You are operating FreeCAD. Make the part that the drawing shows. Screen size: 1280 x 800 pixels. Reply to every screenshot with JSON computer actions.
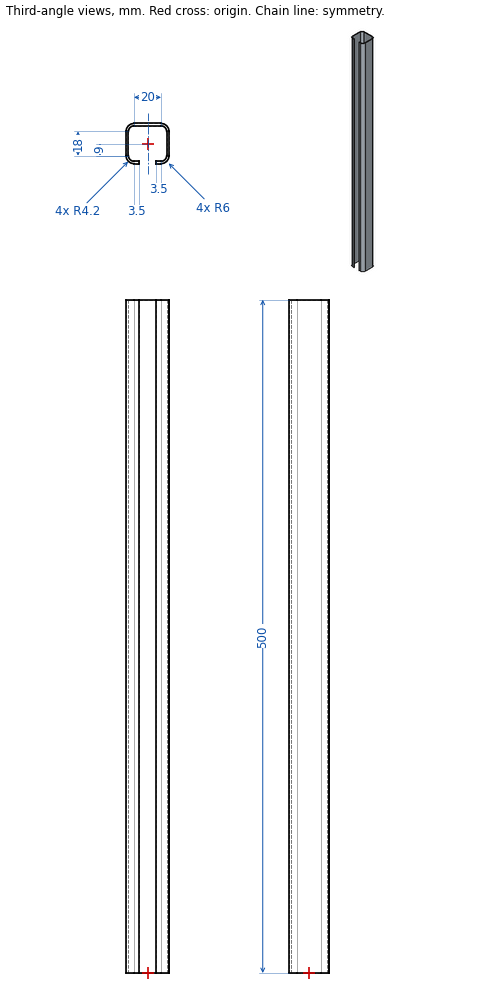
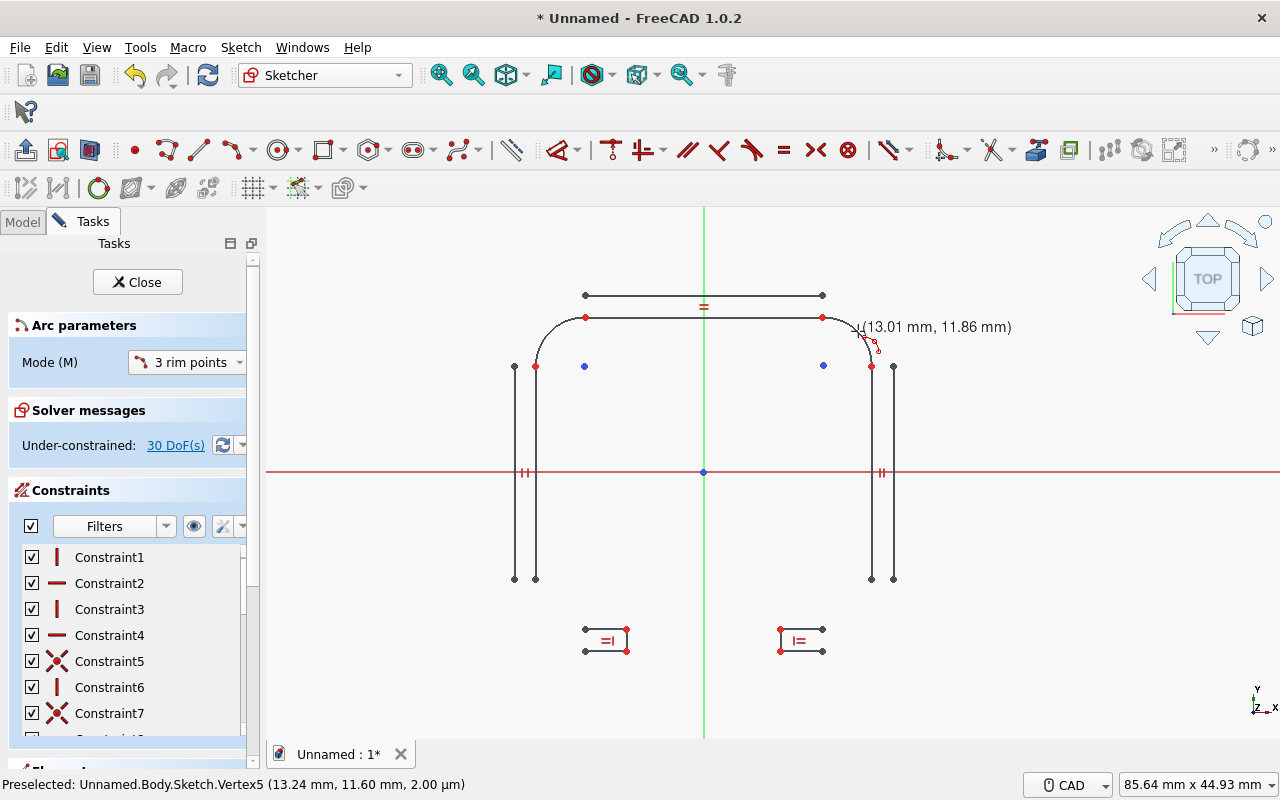
{"action": "left_click", "coordinate": [872, 580]}
{"action": "left_click", "coordinate": [823, 629]}
{"action": "left_click", "coordinate": [858, 614]}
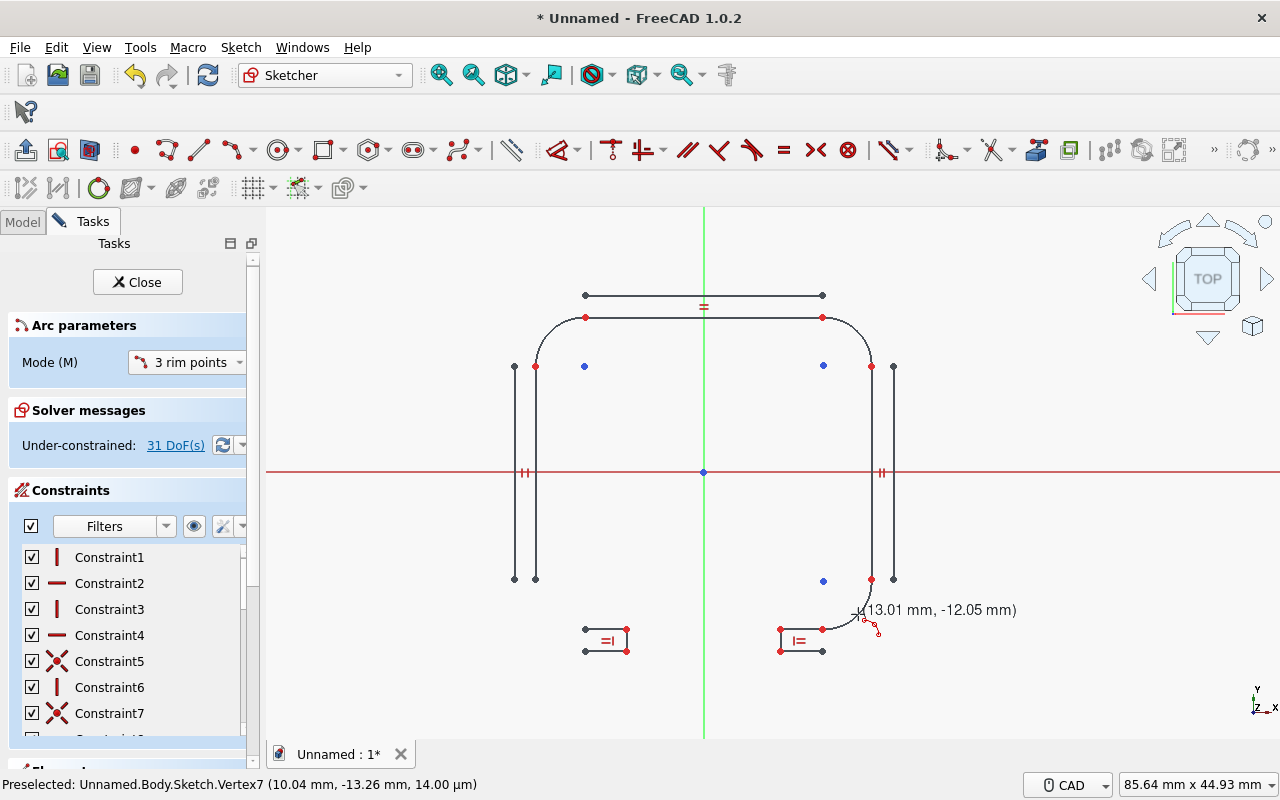
{"action": "left_click", "coordinate": [823, 651]}
{"action": "left_click", "coordinate": [894, 580]}
{"action": "left_click", "coordinate": [873, 629]}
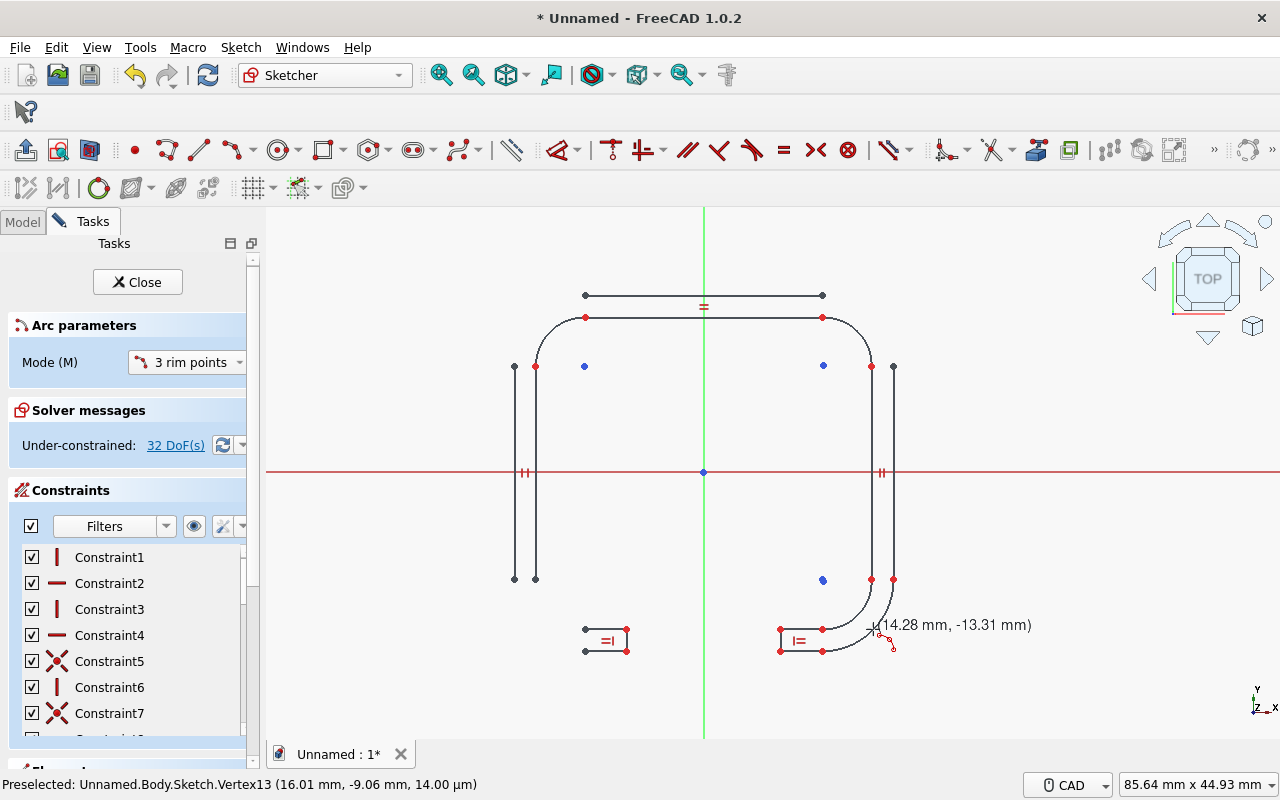
{"action": "left_click", "coordinate": [894, 366]}
{"action": "left_click", "coordinate": [823, 296]}
{"action": "left_click", "coordinate": [873, 316]}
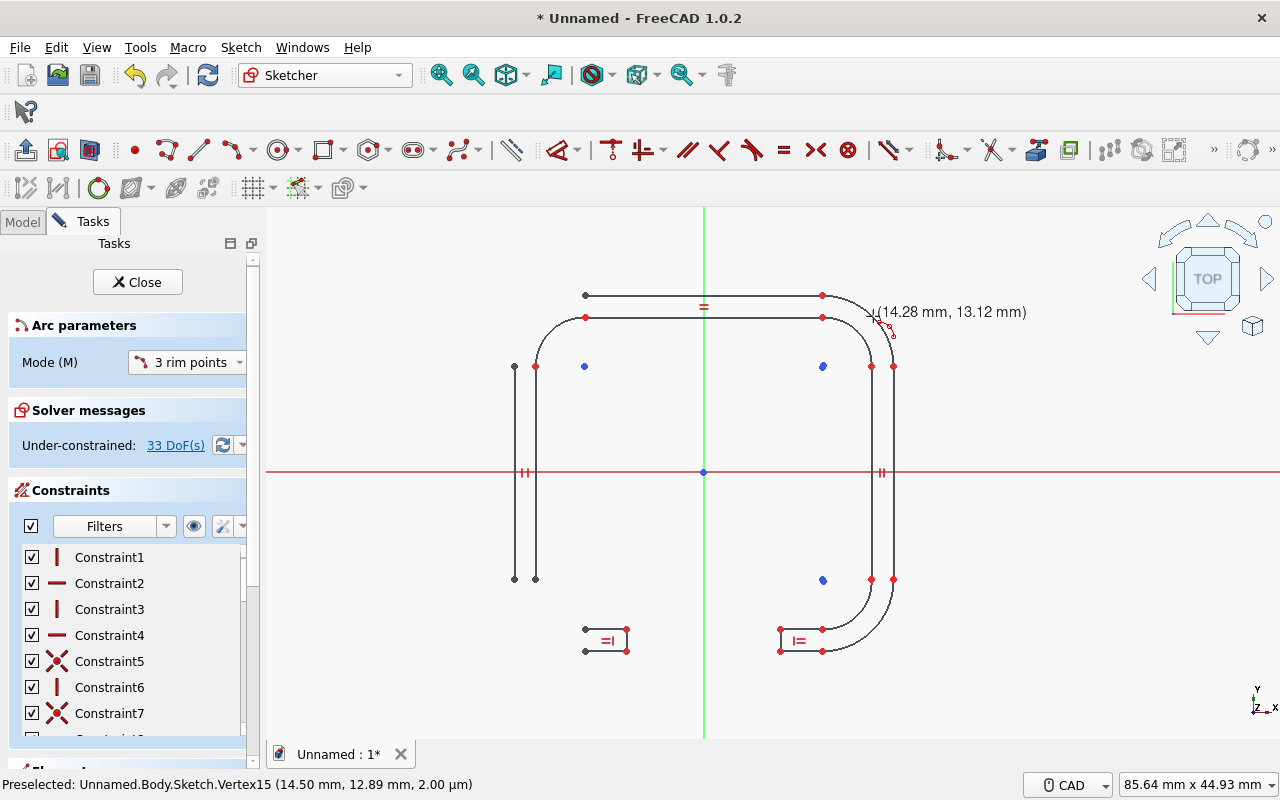
{"action": "left_click", "coordinate": [586, 296]}
{"action": "left_click", "coordinate": [515, 366]}
{"action": "left_click", "coordinate": [535, 316]}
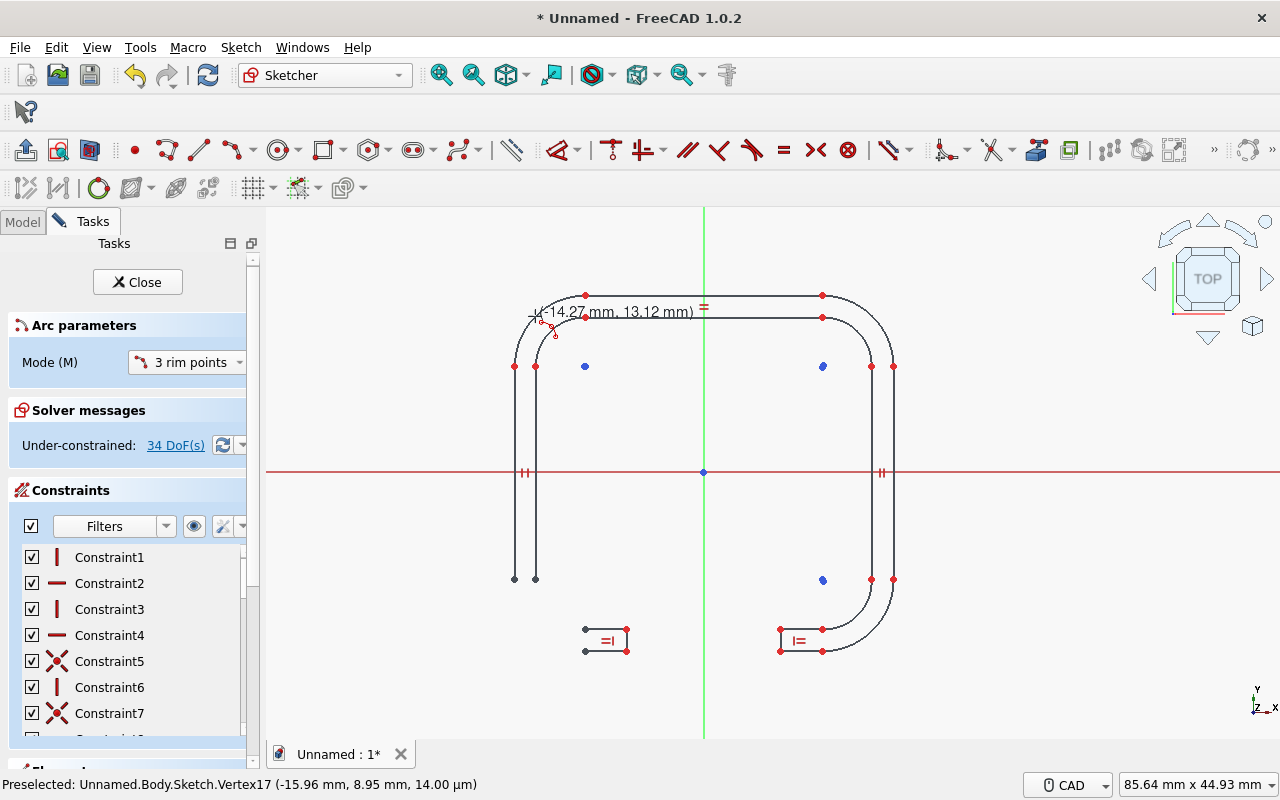
{"action": "left_click", "coordinate": [515, 580]}
{"action": "left_click", "coordinate": [586, 651]}
{"action": "left_click", "coordinate": [535, 629]}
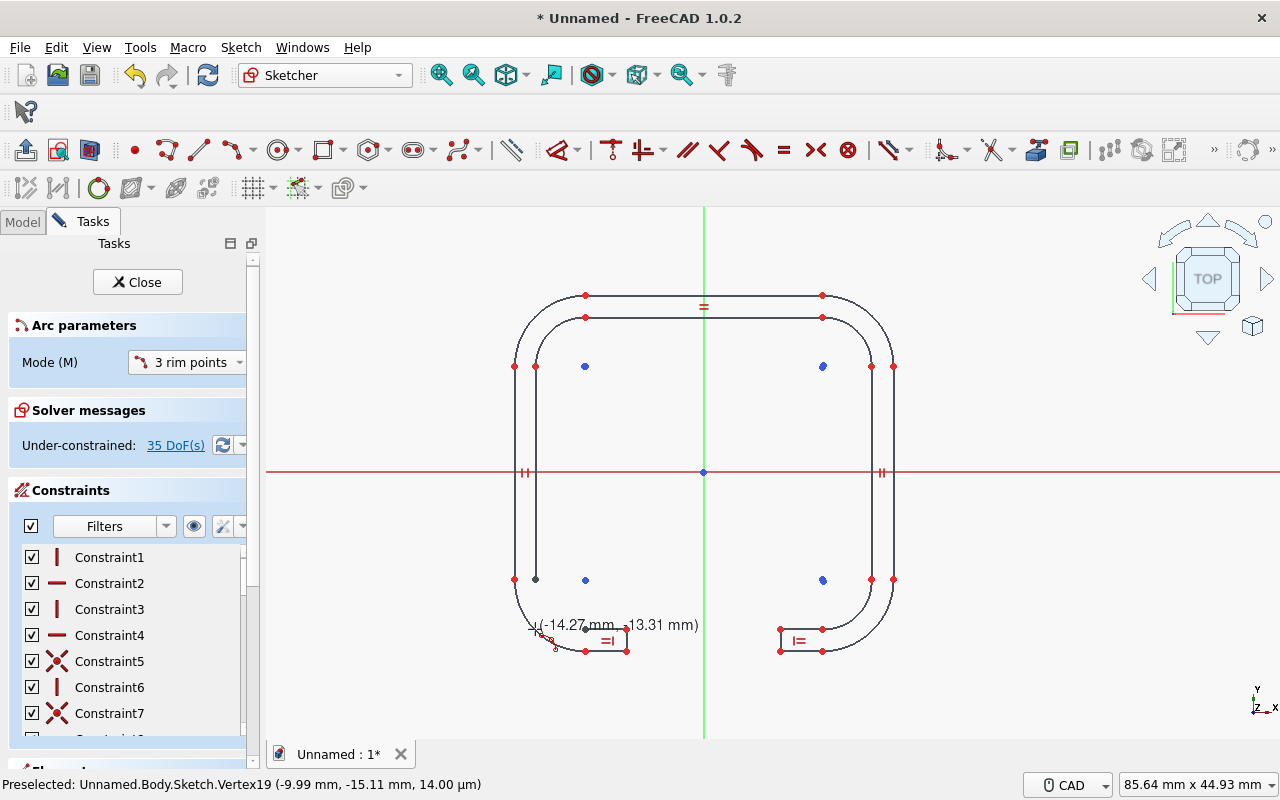
{"action": "left_click", "coordinate": [586, 629]}
{"action": "left_click", "coordinate": [536, 580]}
{"action": "left_click", "coordinate": [550, 614]}
{"action": "key", "text": "Escape"}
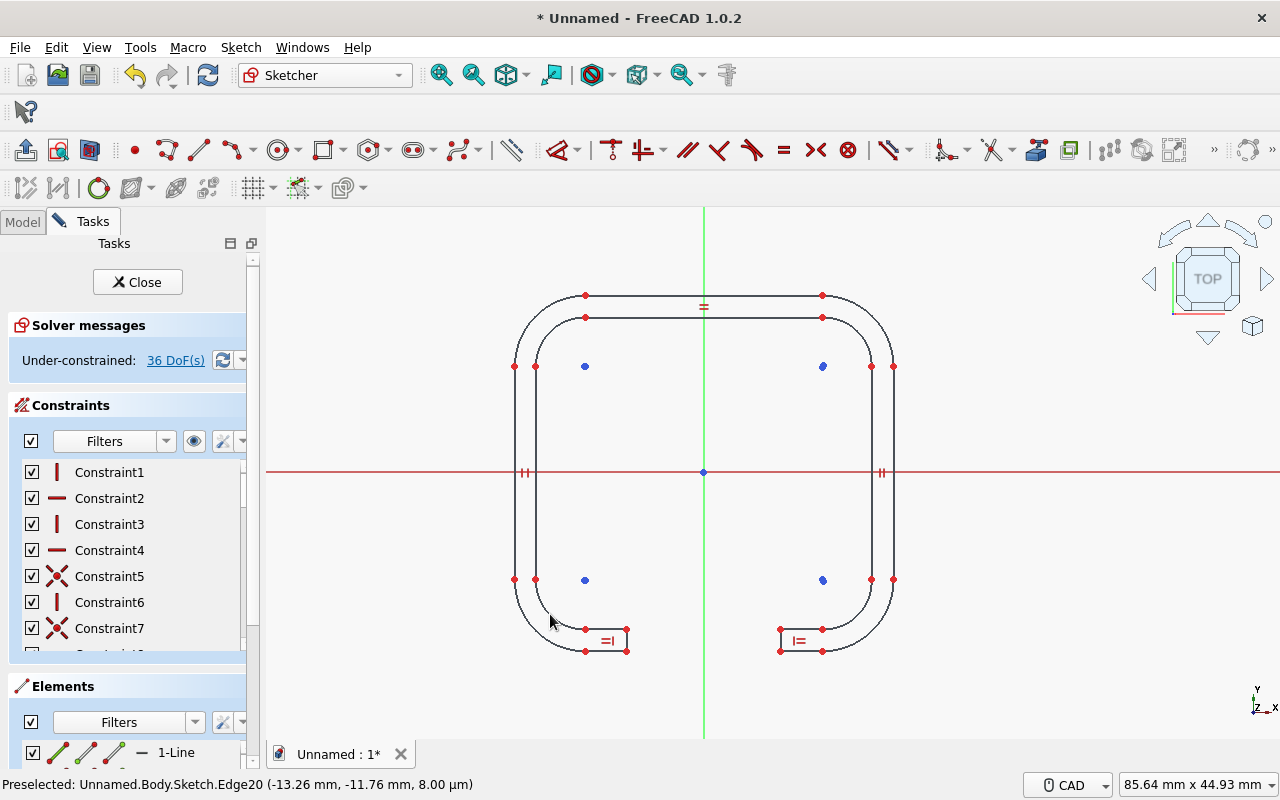
{"action": "left_click", "coordinate": [536, 516]}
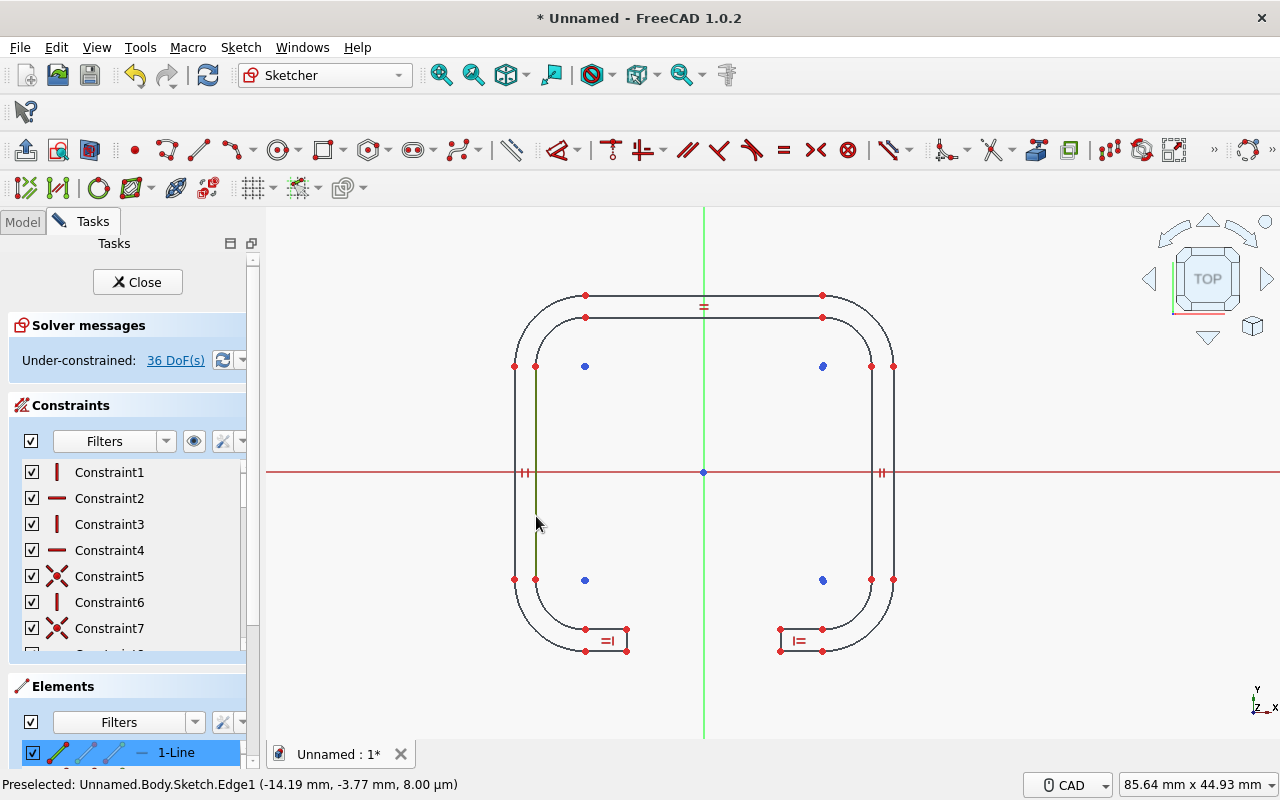
{"action": "left_click", "coordinate": [563, 323]}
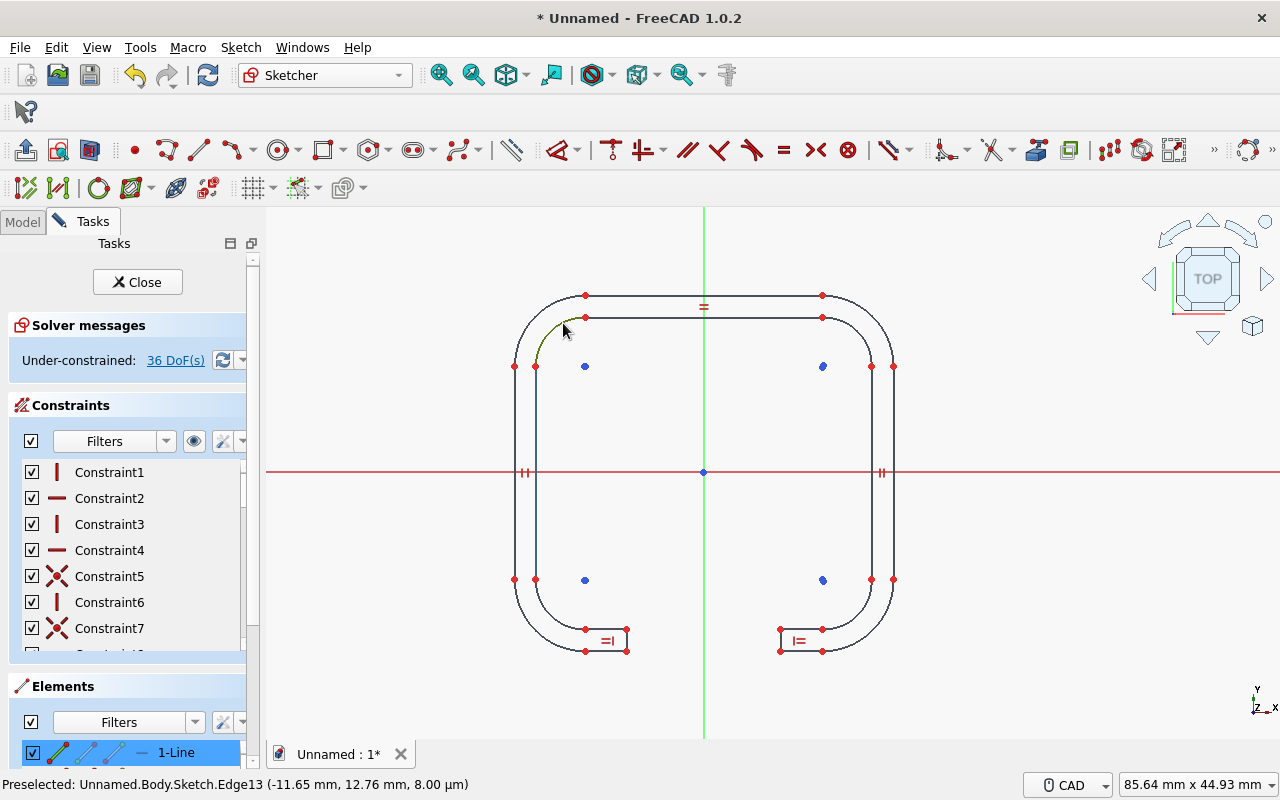
{"action": "left_click", "coordinate": [752, 150]}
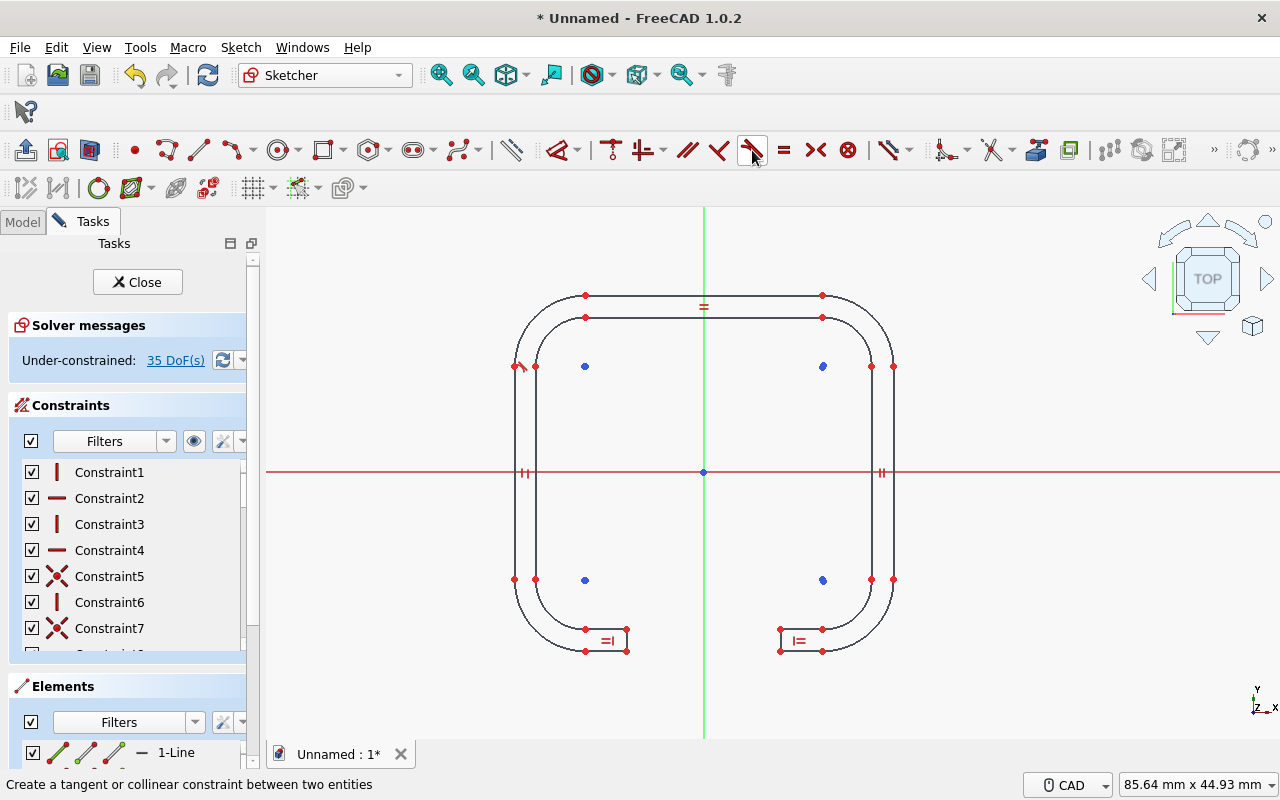
{"action": "left_click", "coordinate": [536, 516]}